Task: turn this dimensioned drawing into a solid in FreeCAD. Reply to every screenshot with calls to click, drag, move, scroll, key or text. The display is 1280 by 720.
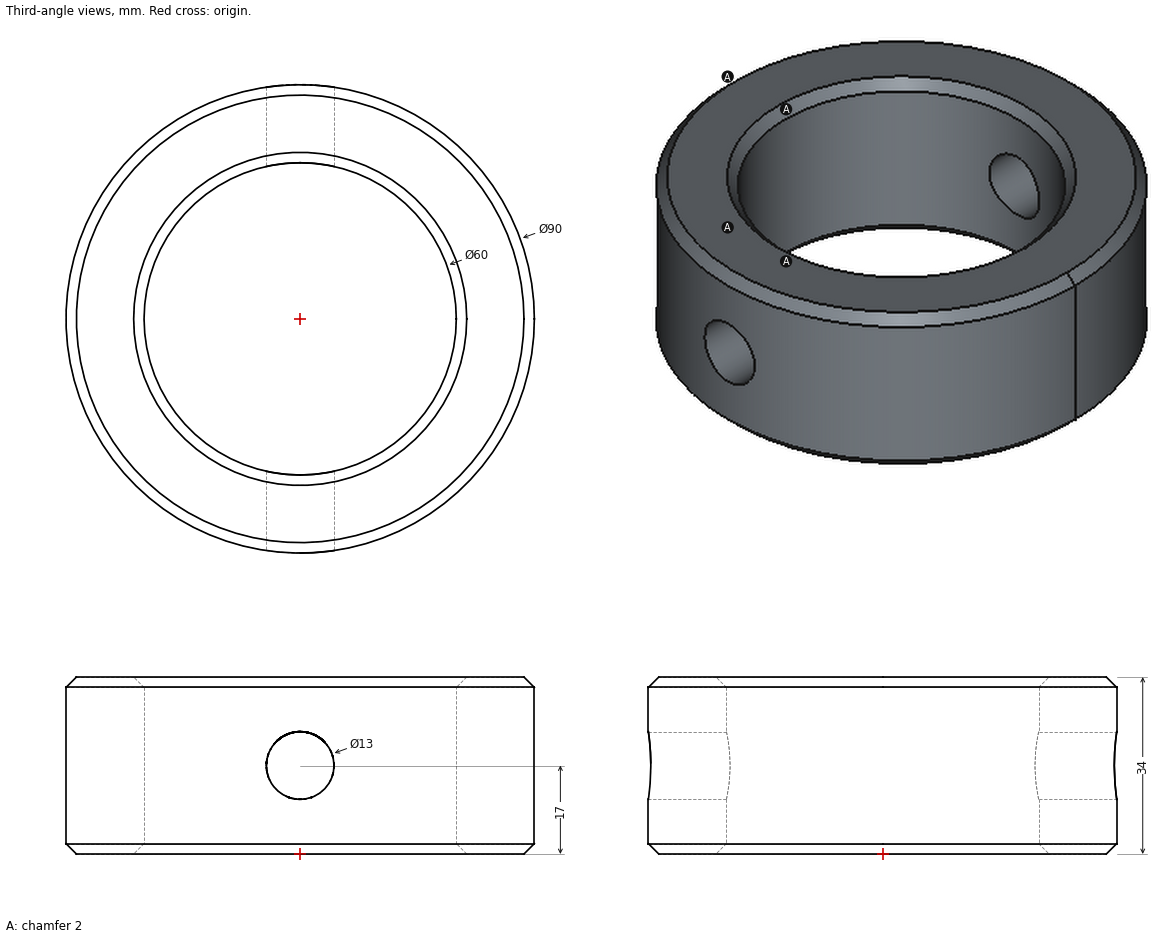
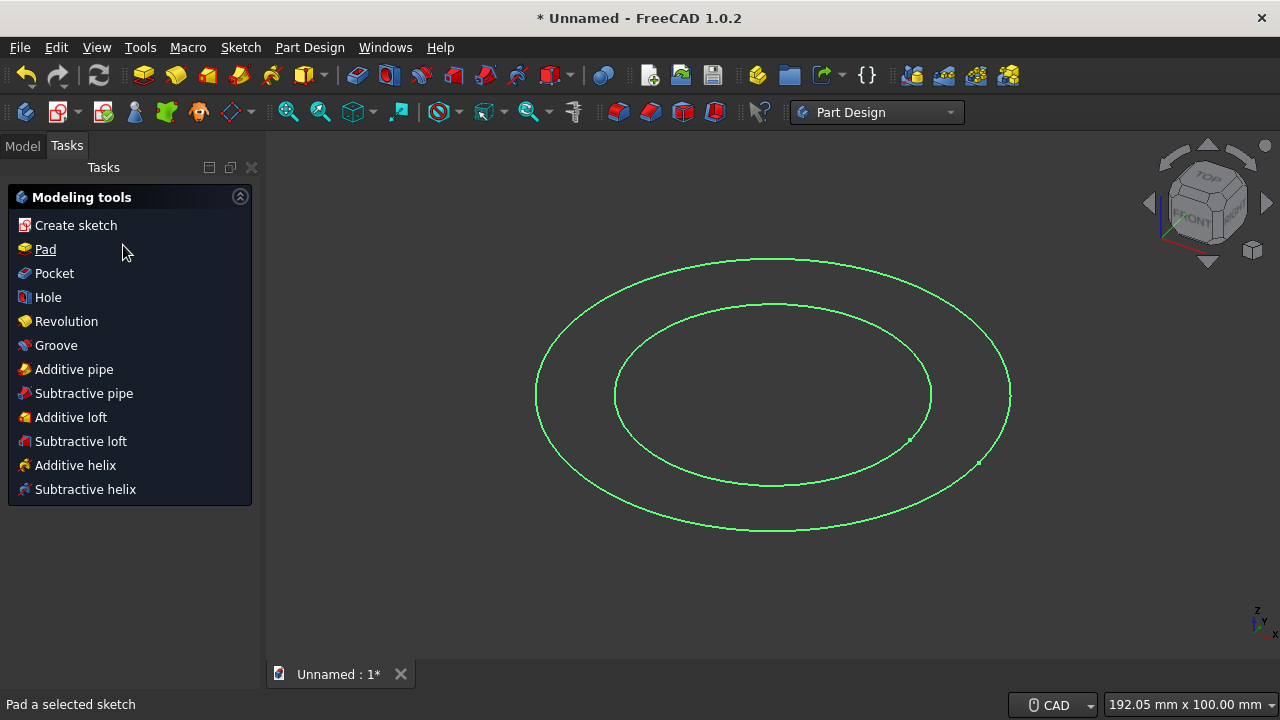
click(144, 76)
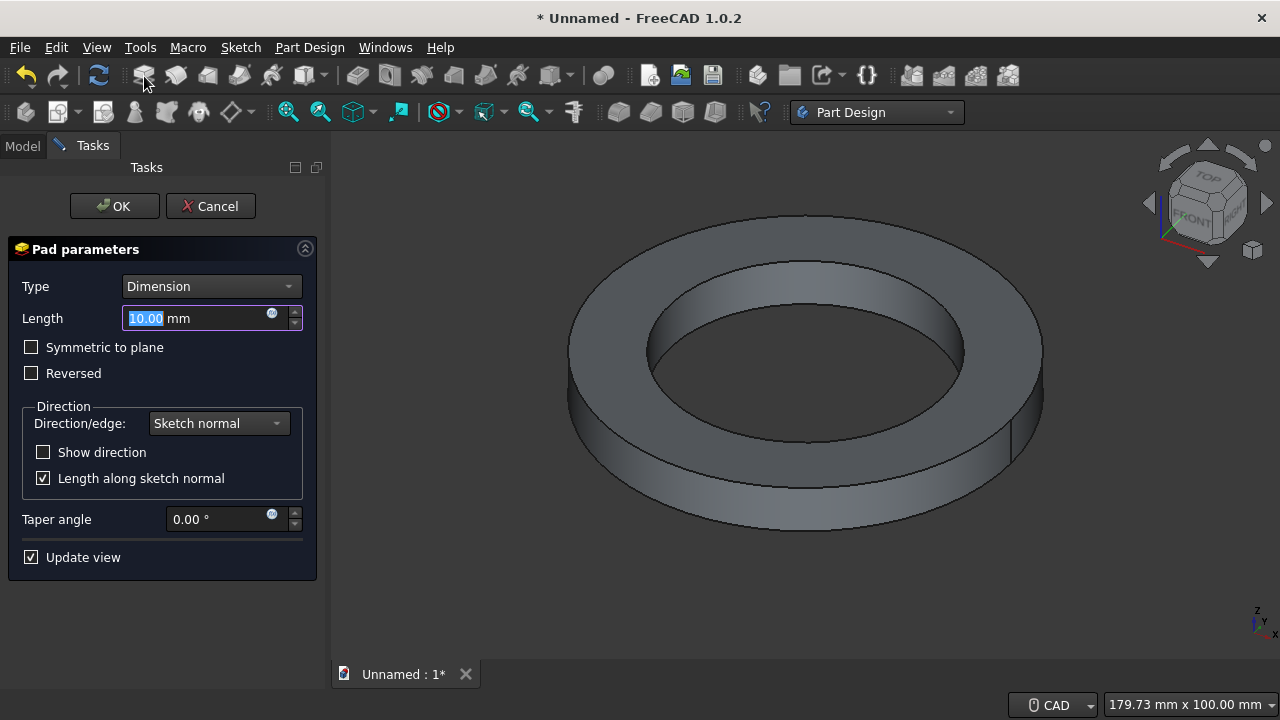
text(34)
key(Tab)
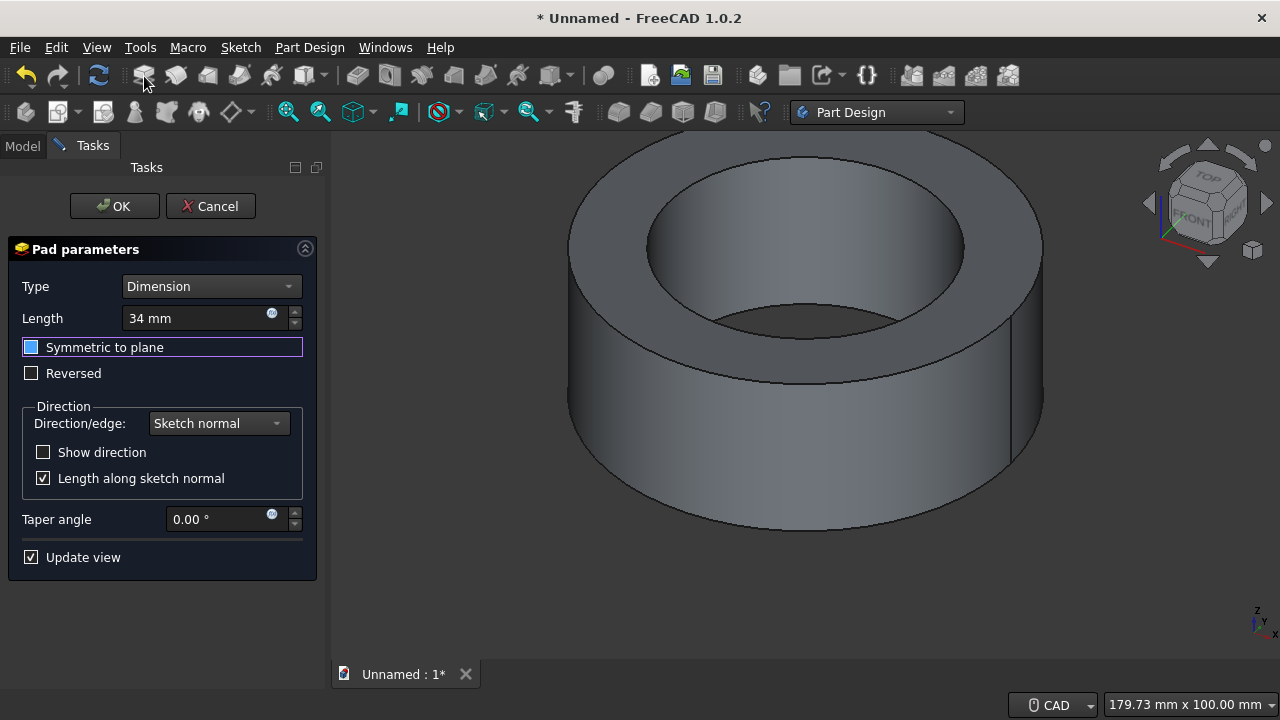
click(115, 206)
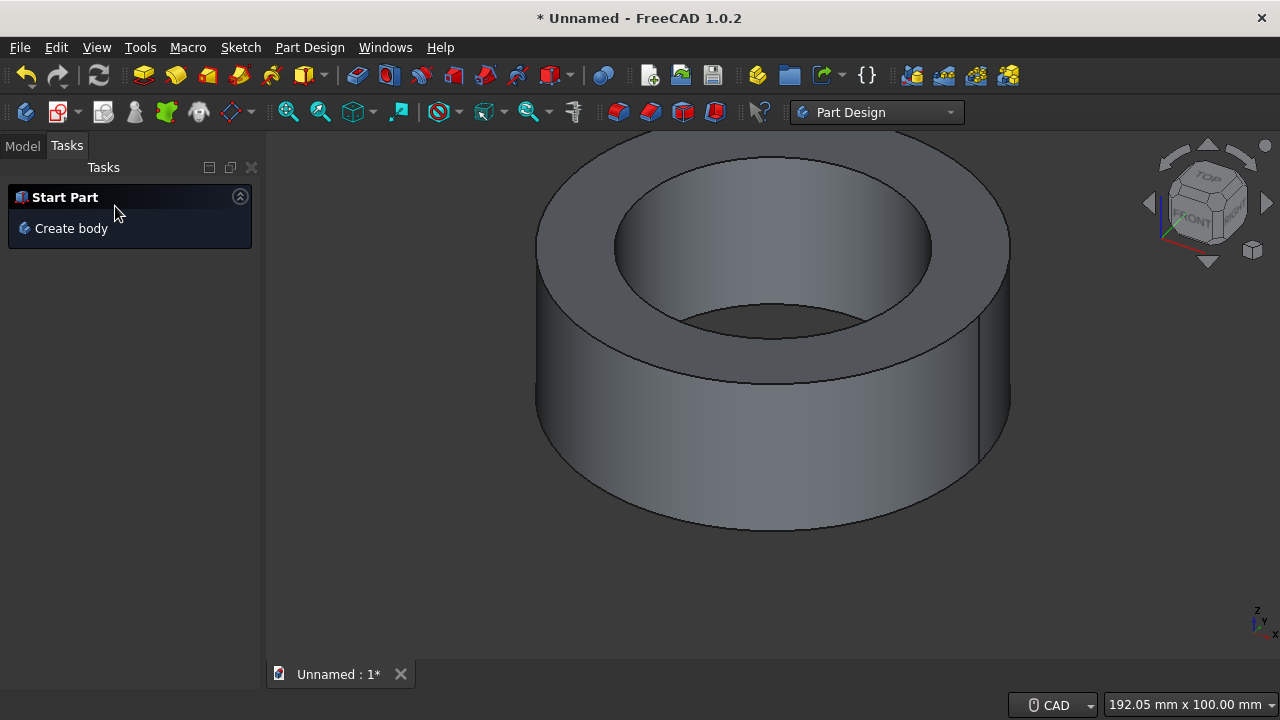
click(290, 112)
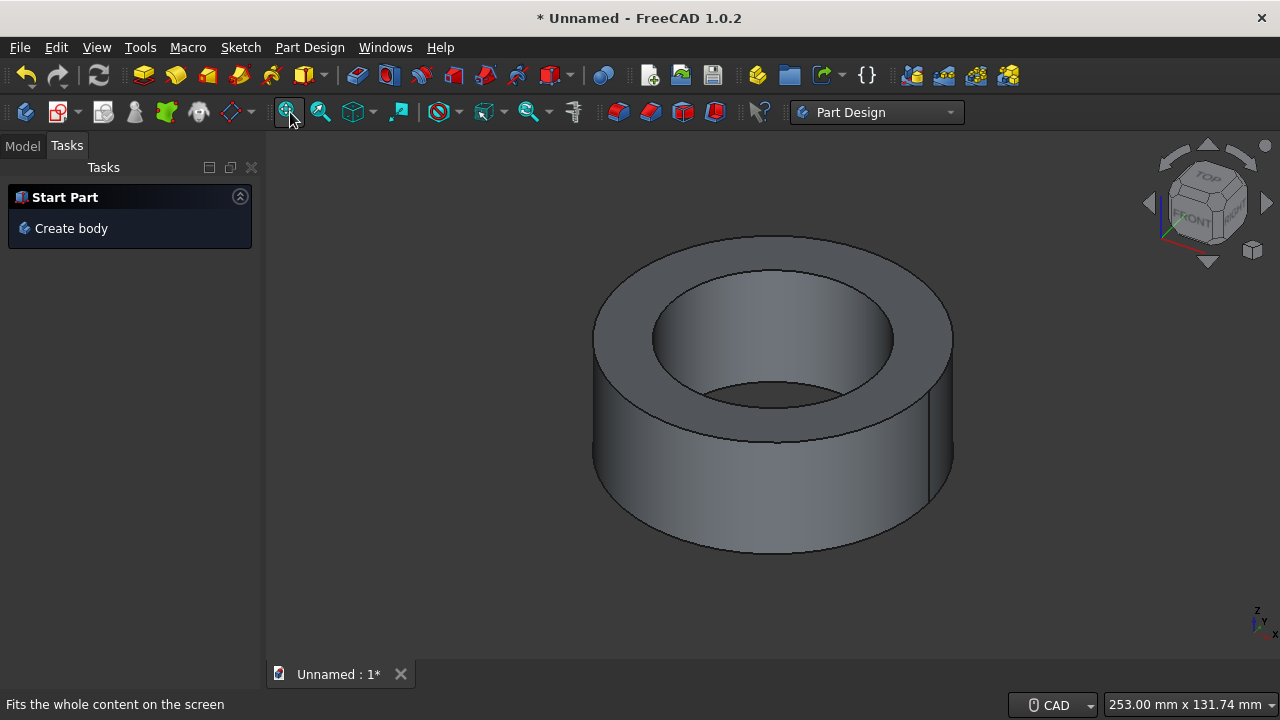
click(58, 112)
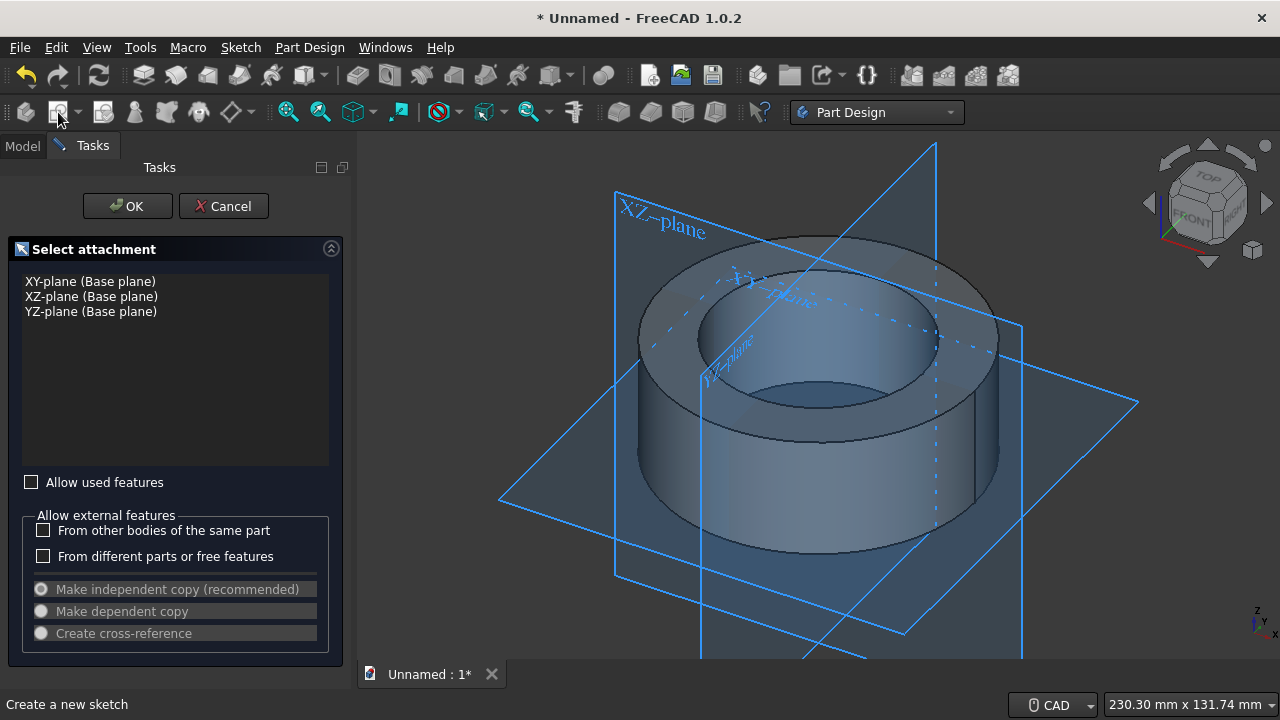
click(82, 296)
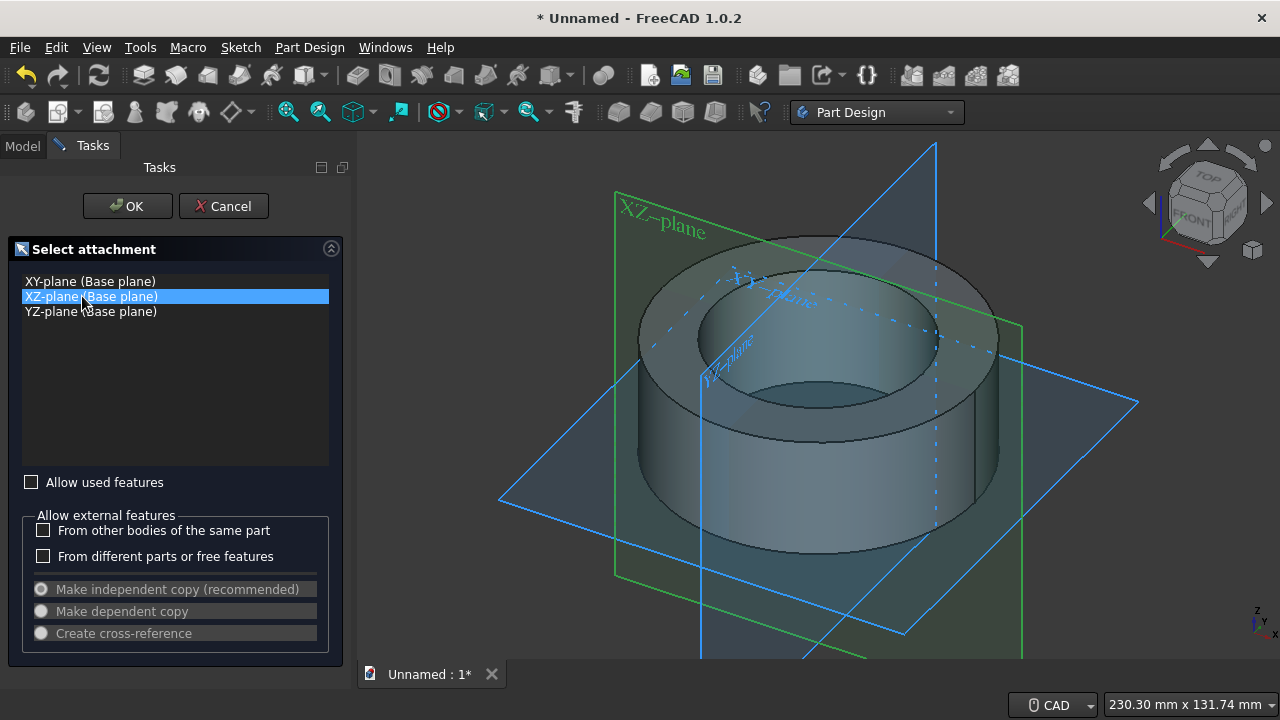
click(128, 206)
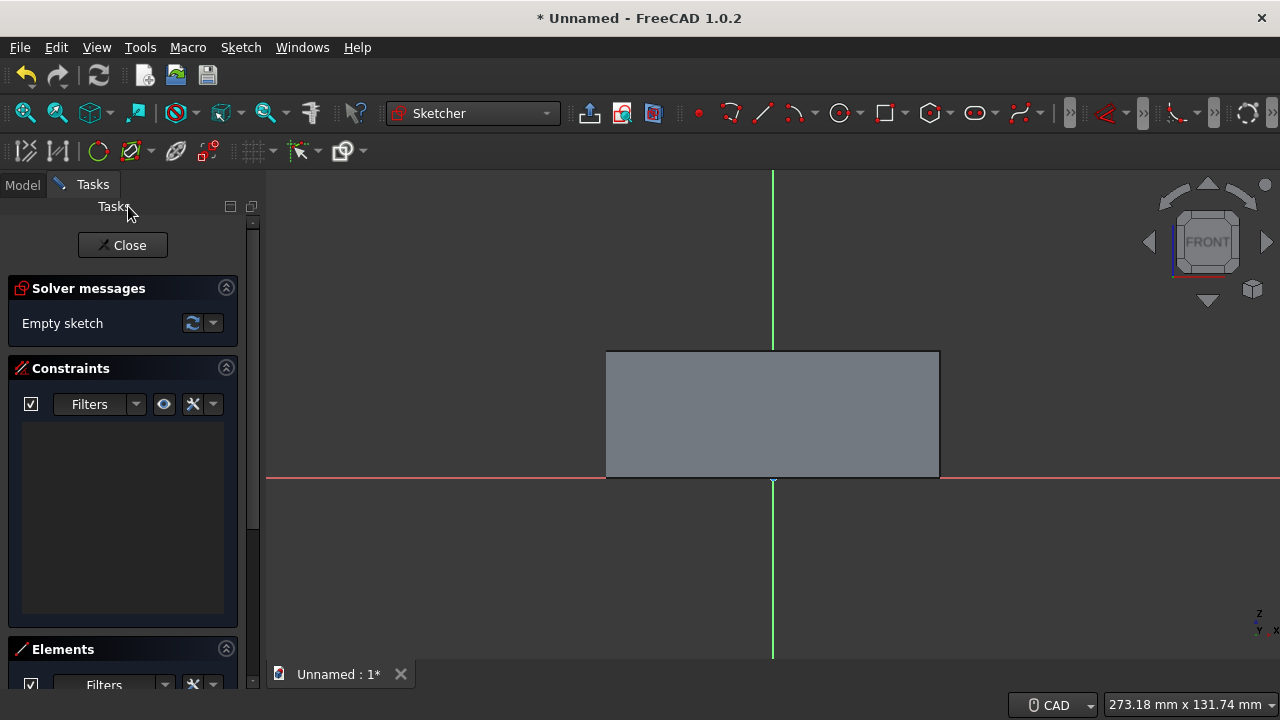
key(q)
key(s)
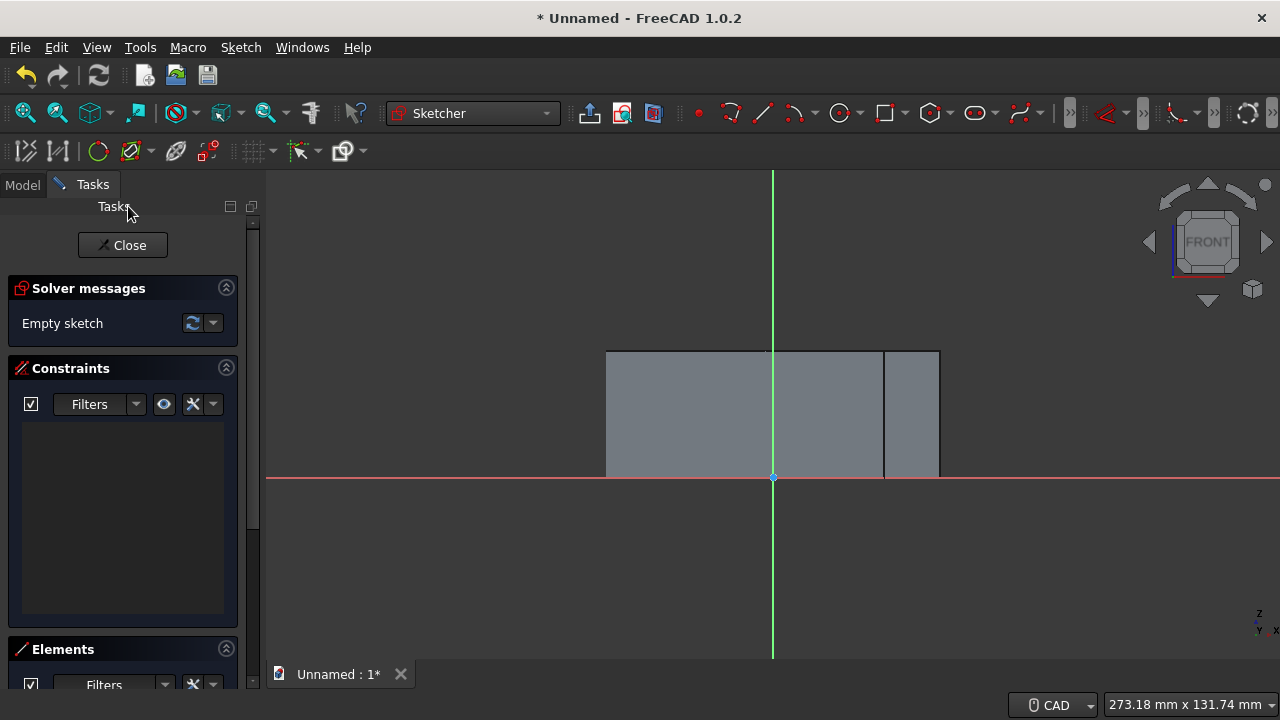
scroll(803, 442, up, 6)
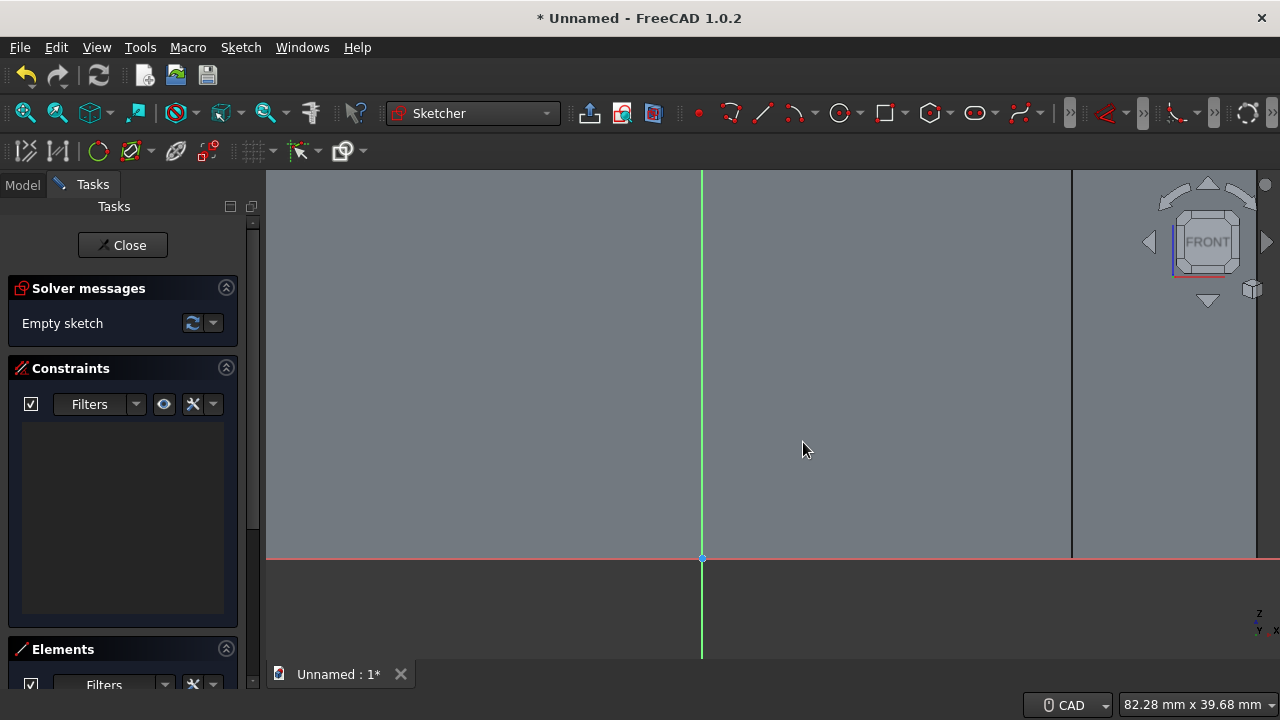
click(840, 114)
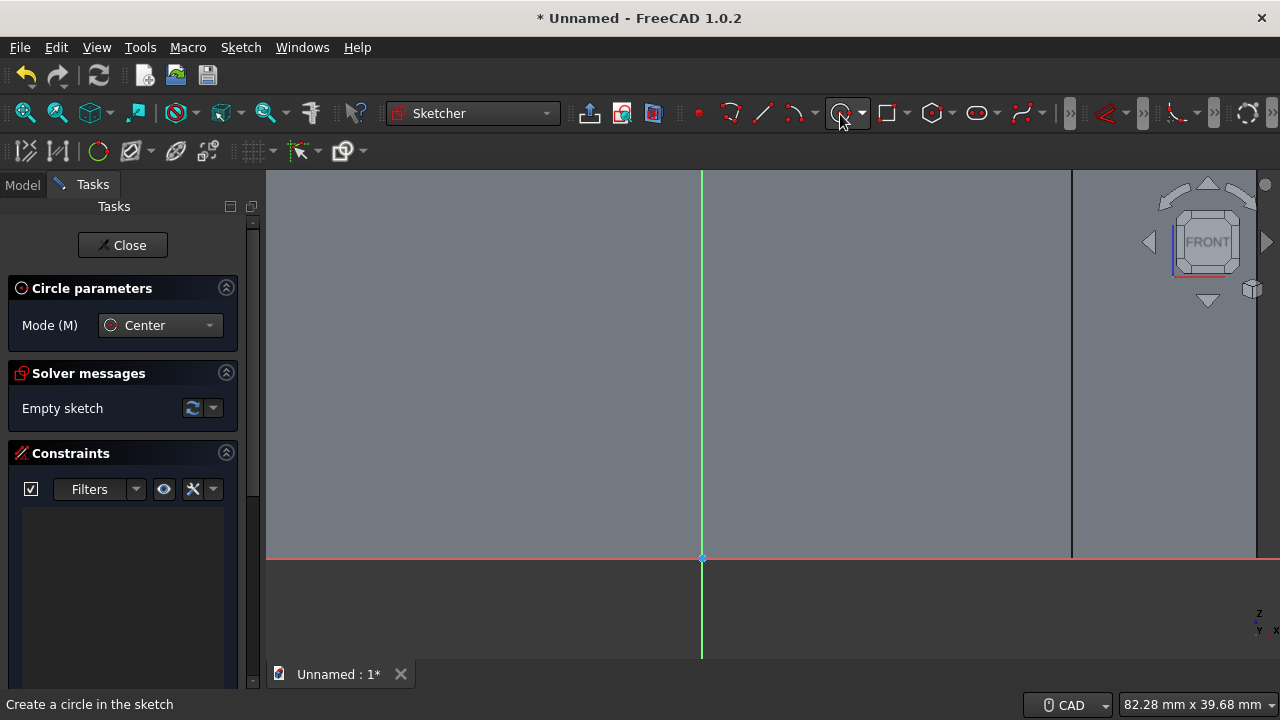
click(702, 349)
move(759, 293)